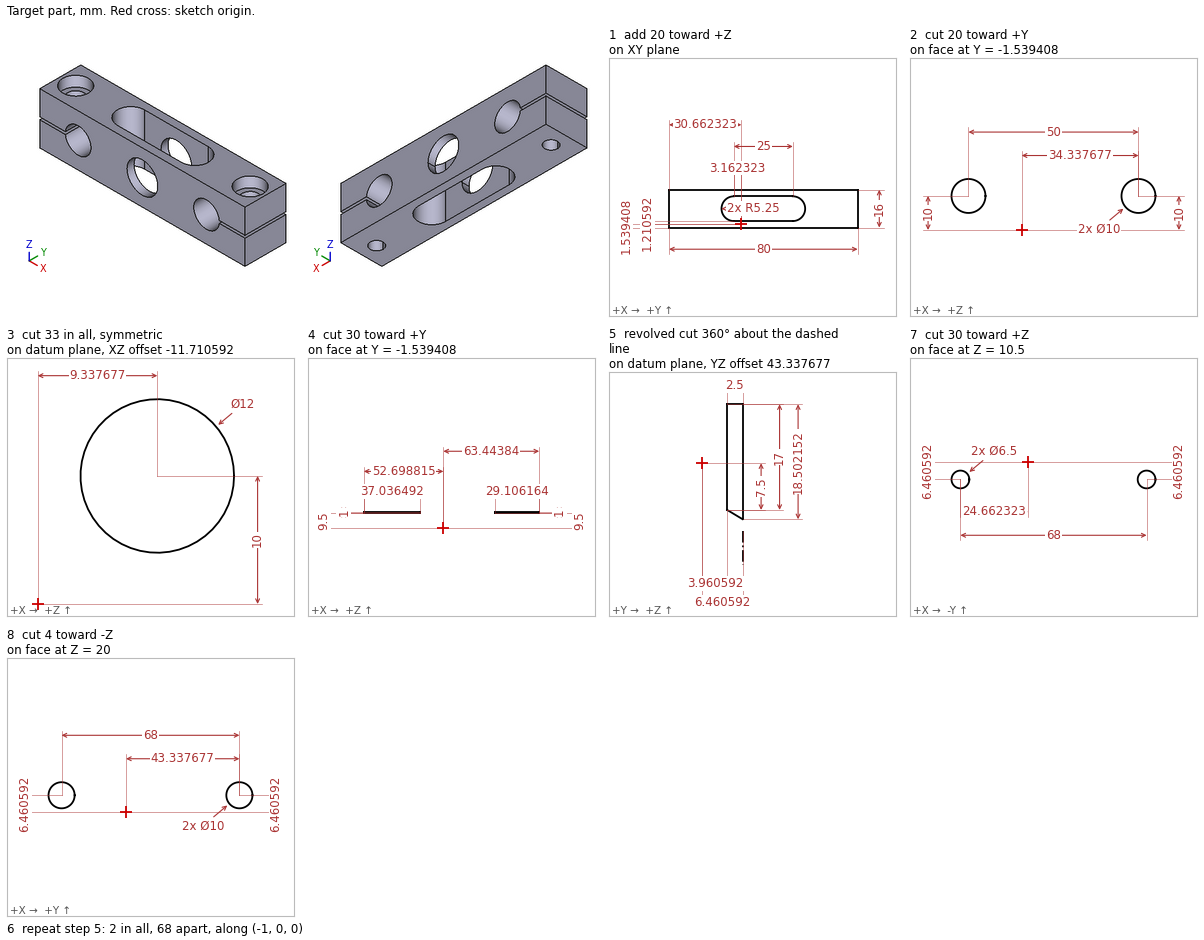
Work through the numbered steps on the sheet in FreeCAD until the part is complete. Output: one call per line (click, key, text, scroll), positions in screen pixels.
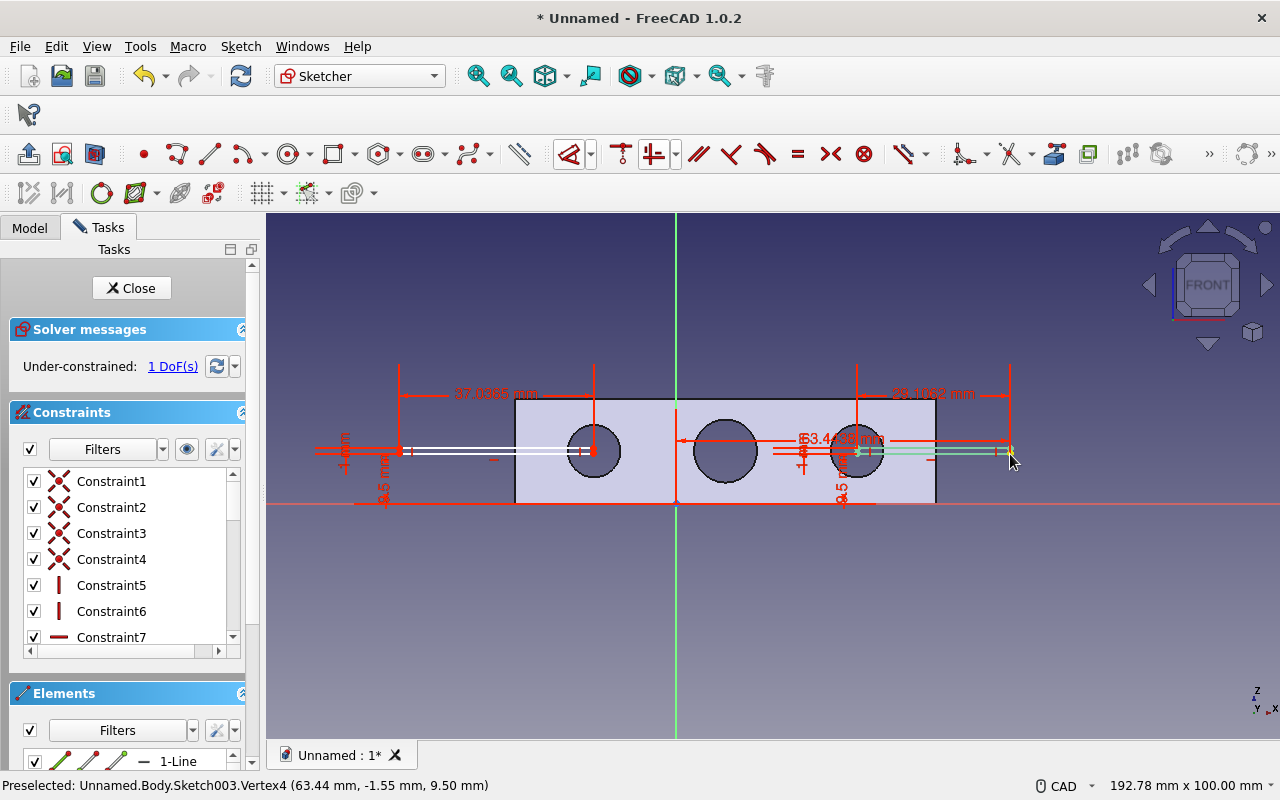
scroll(399, 448, up, 5)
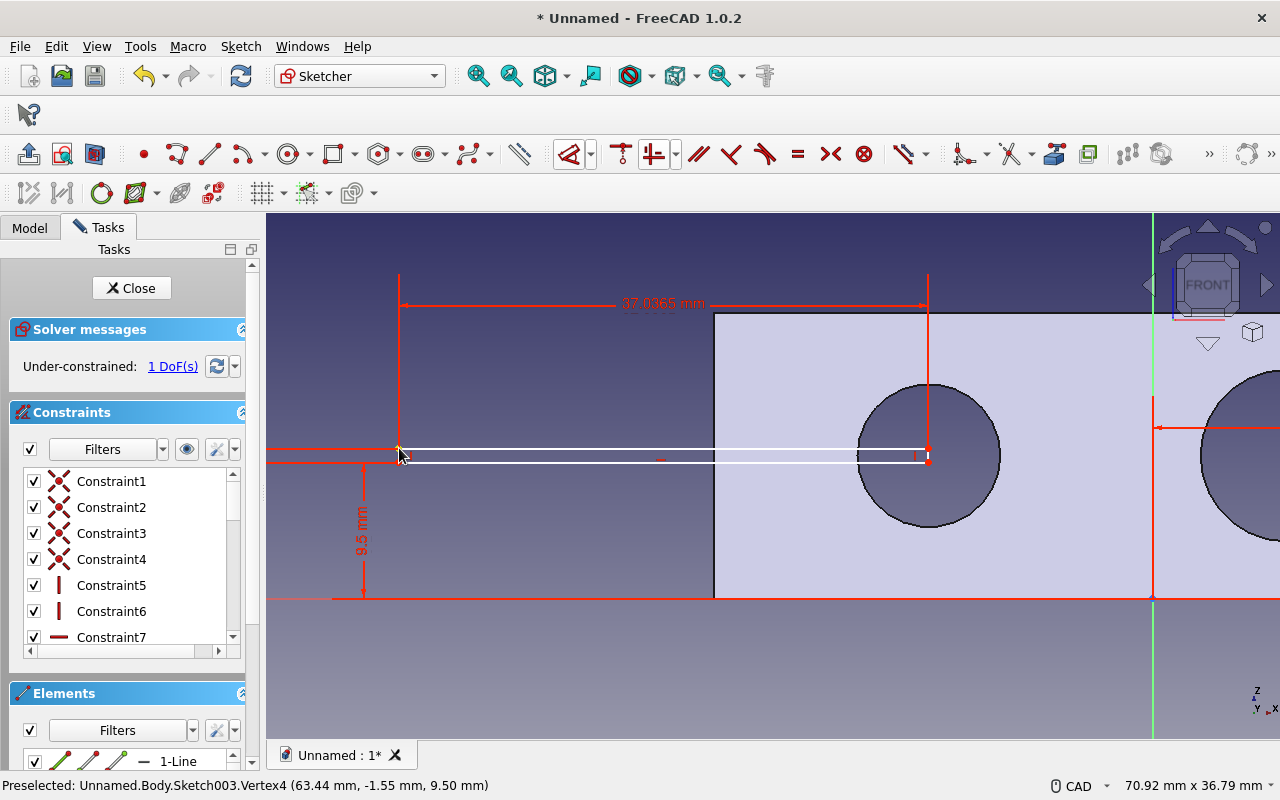
click(399, 449)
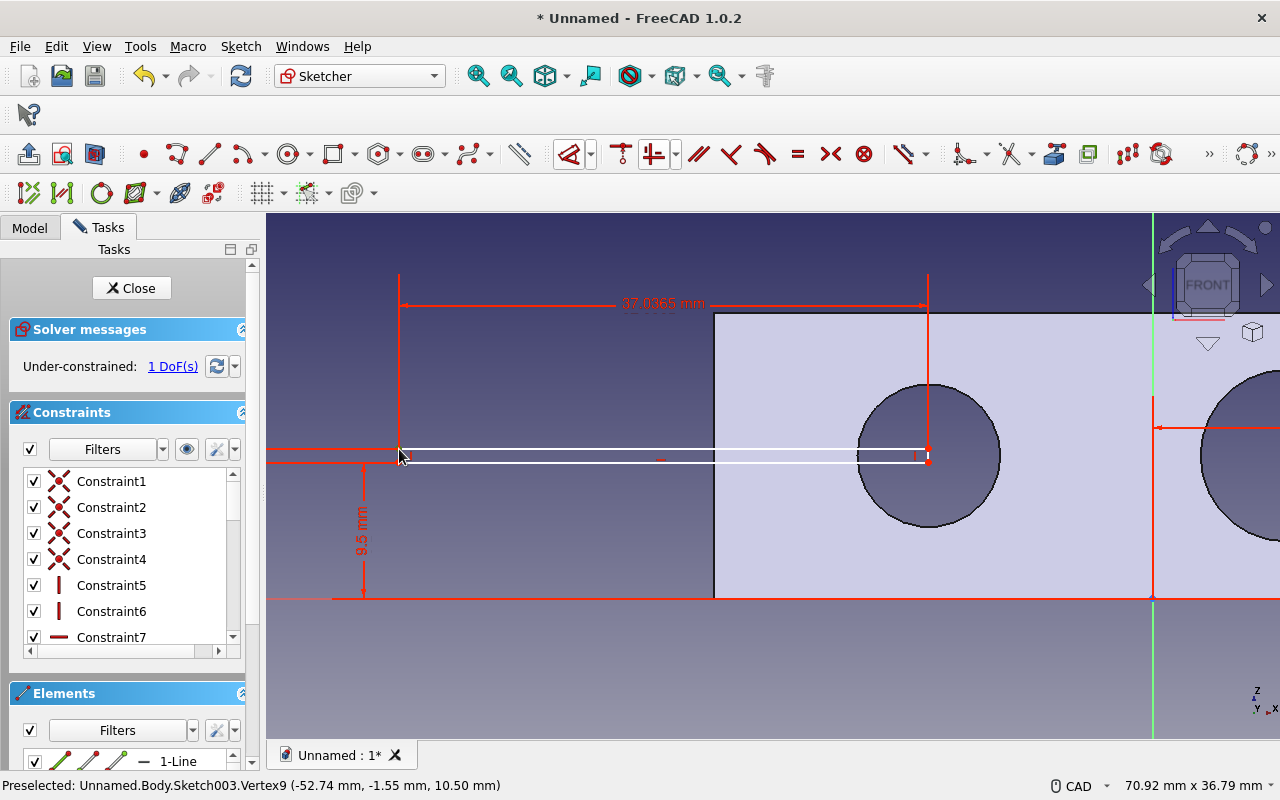
key(l)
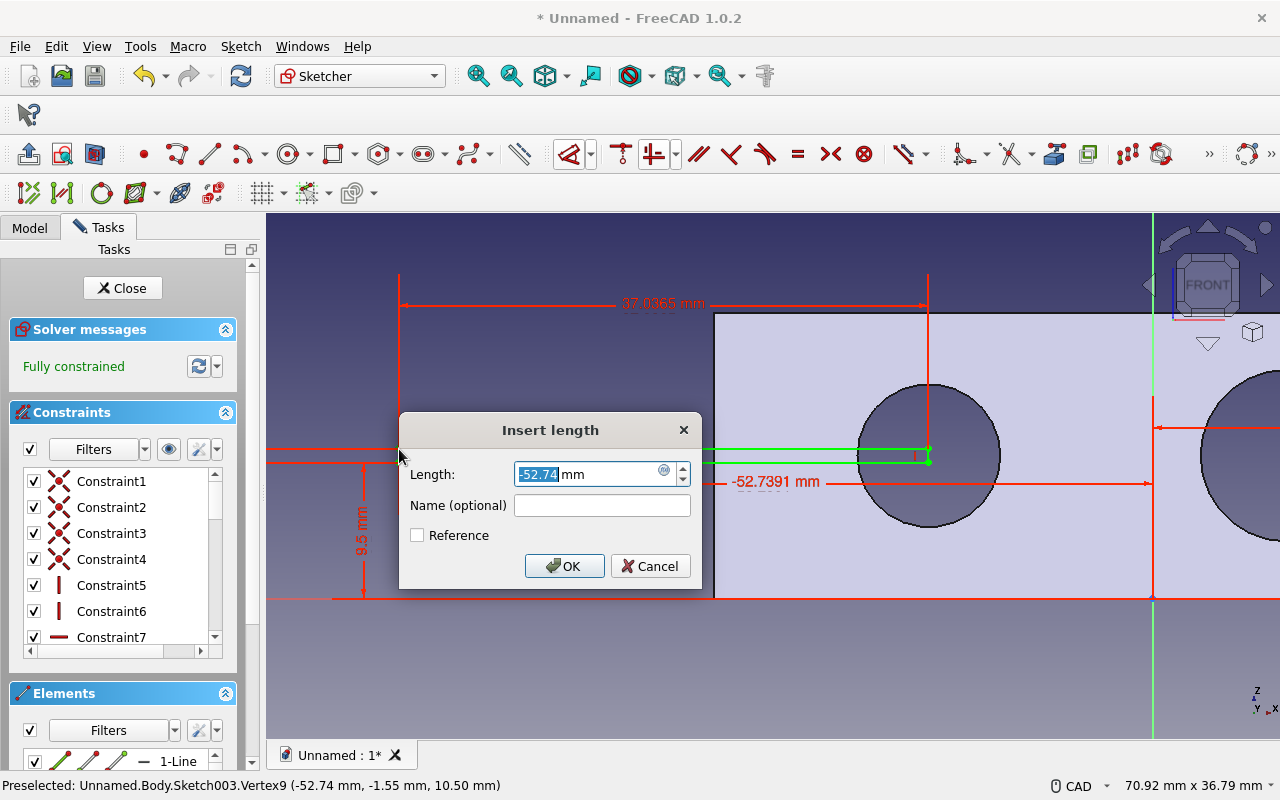
text(-52.698815)
key(Return)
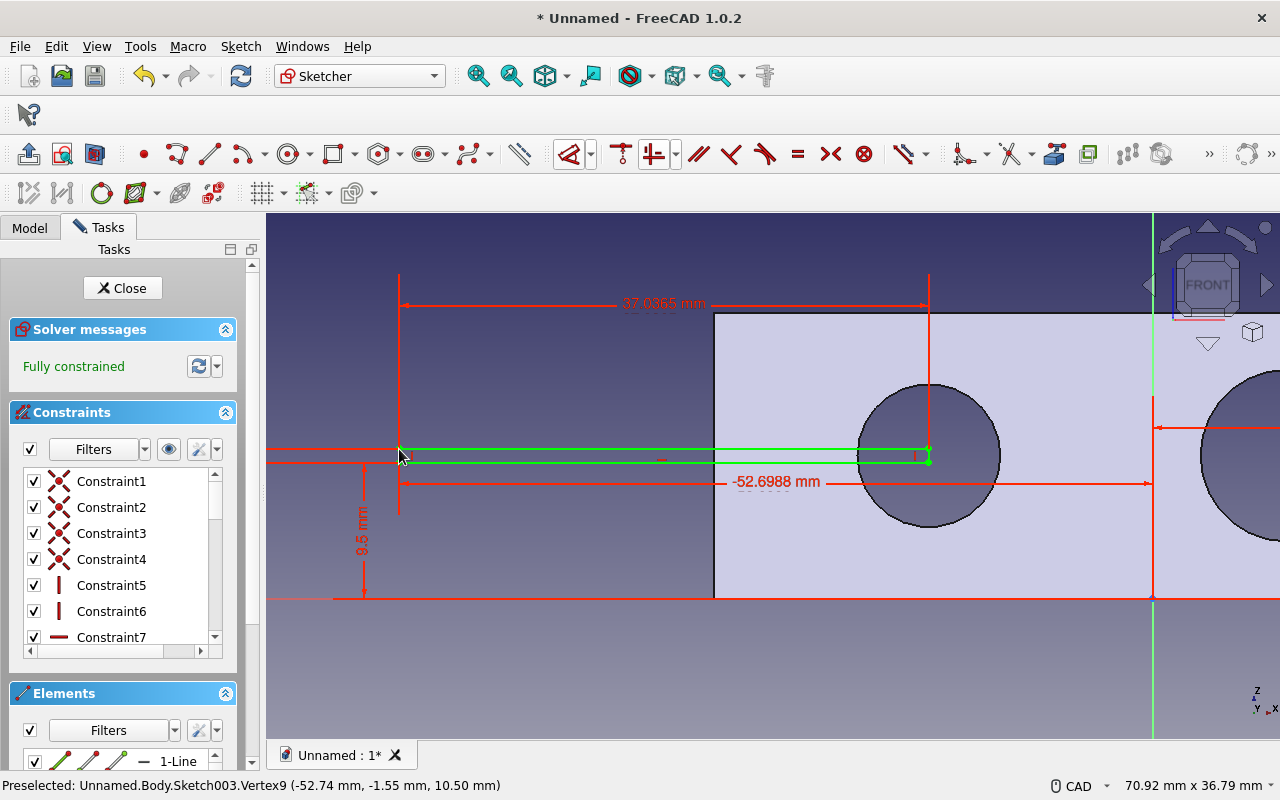
click(123, 288)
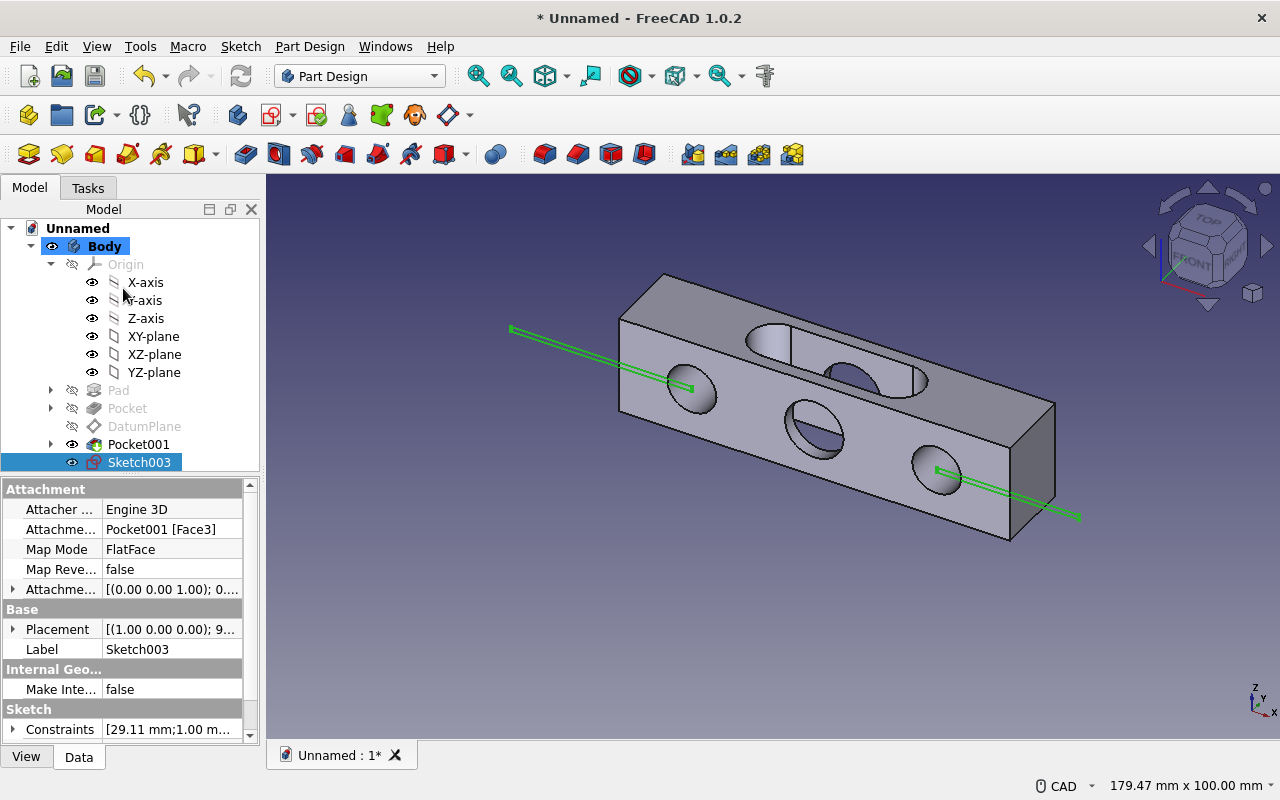
click(246, 154)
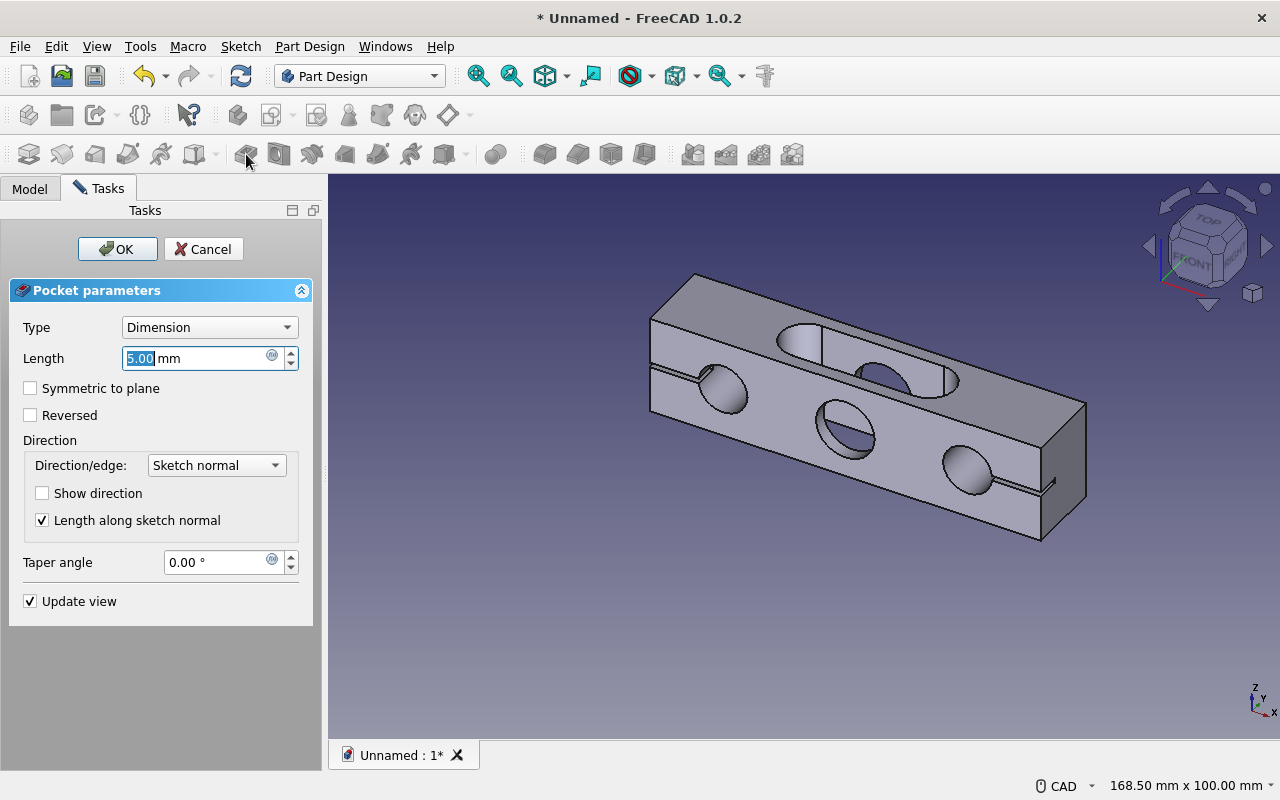
text(30)
key(Tab)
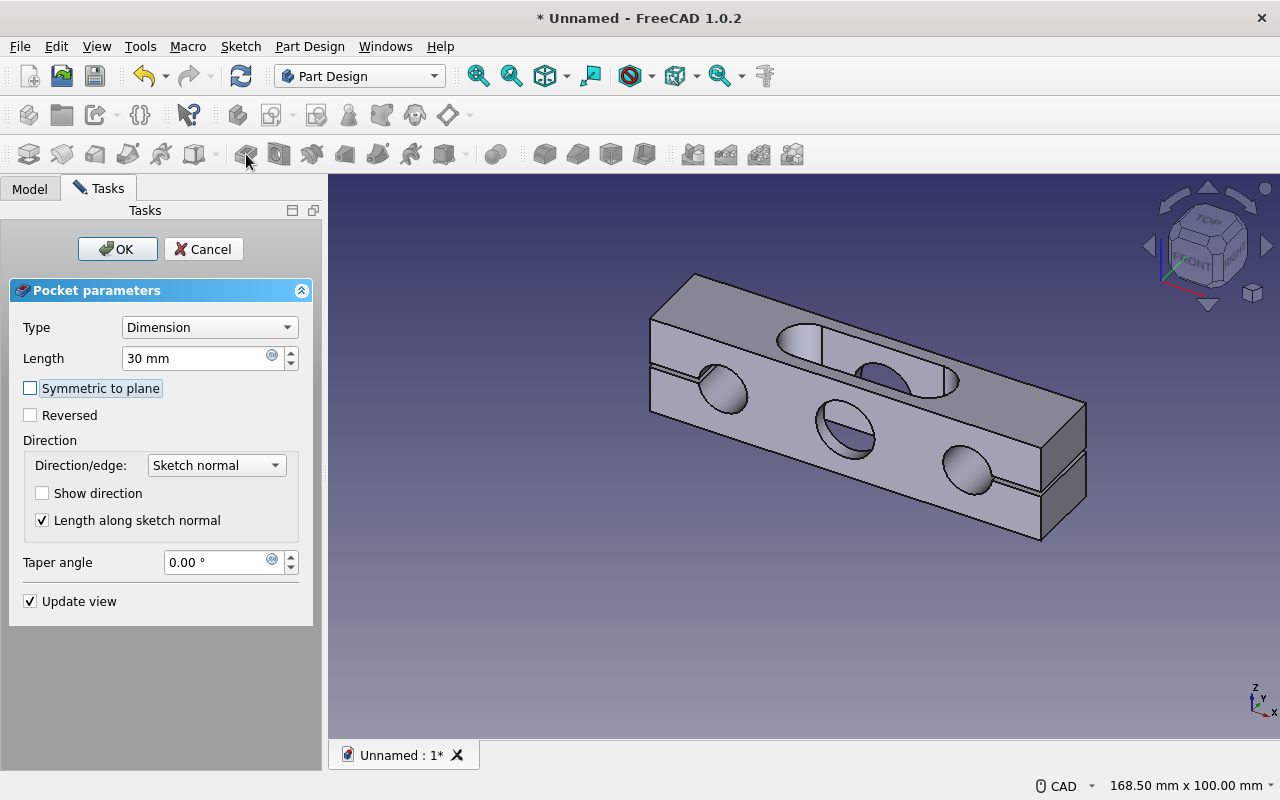
click(118, 249)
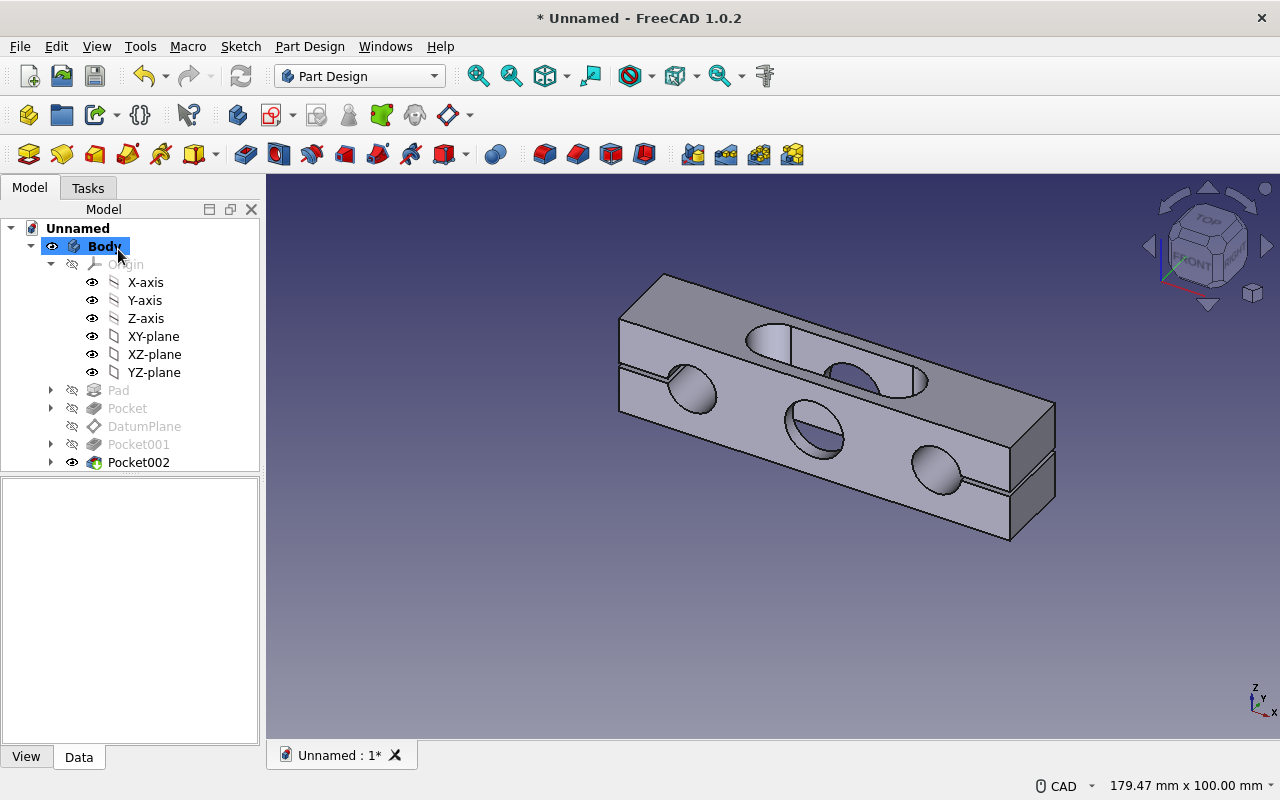
click(137, 372)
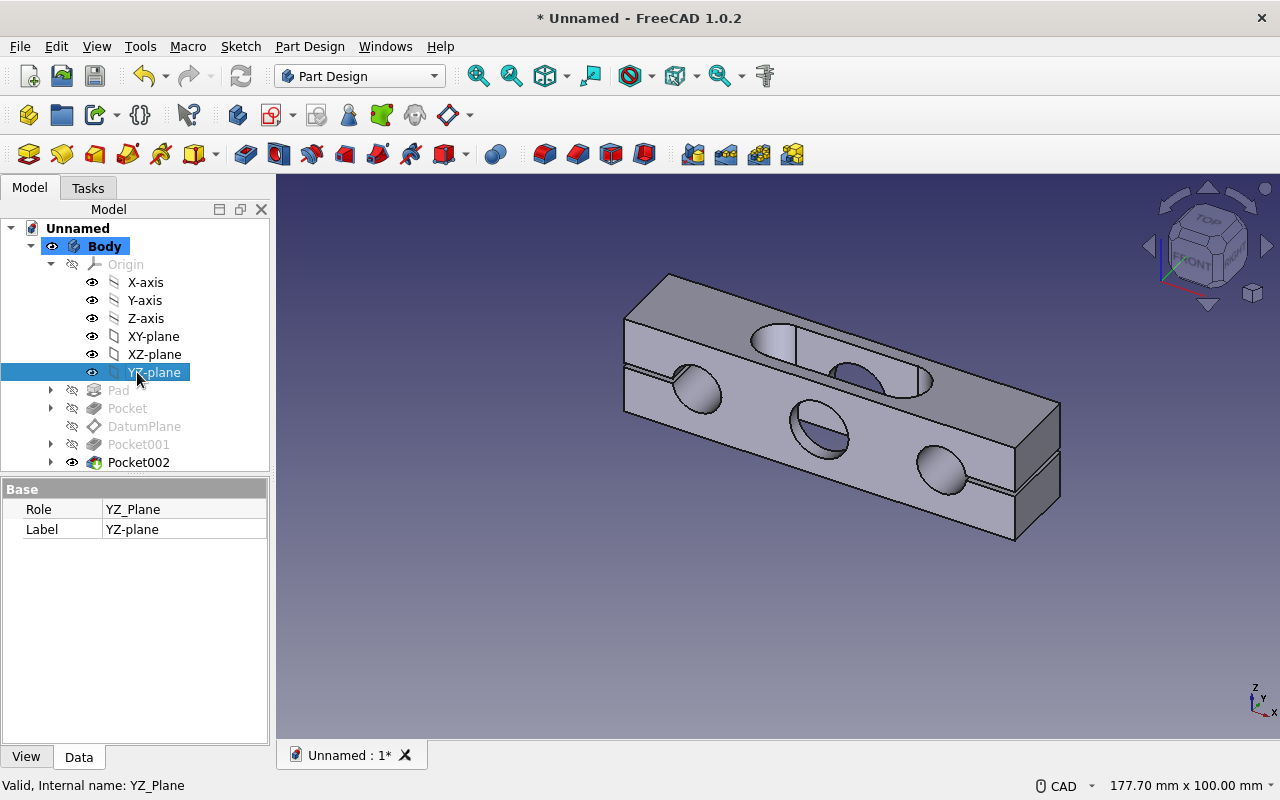
click(448, 116)